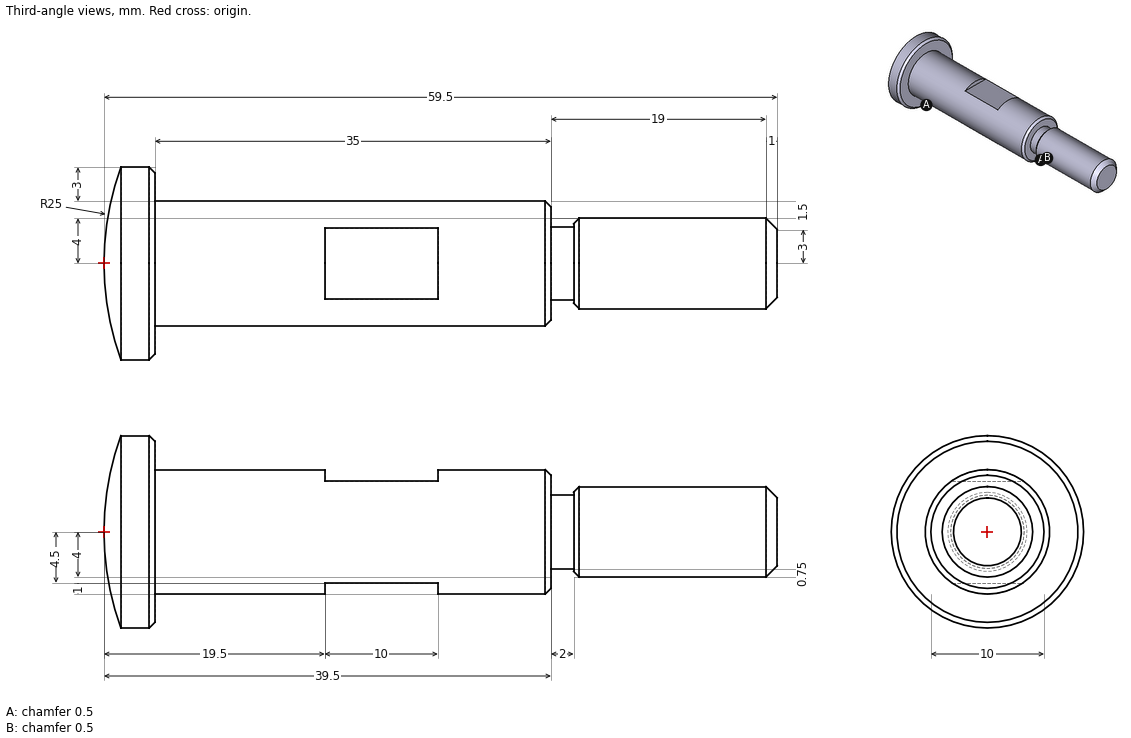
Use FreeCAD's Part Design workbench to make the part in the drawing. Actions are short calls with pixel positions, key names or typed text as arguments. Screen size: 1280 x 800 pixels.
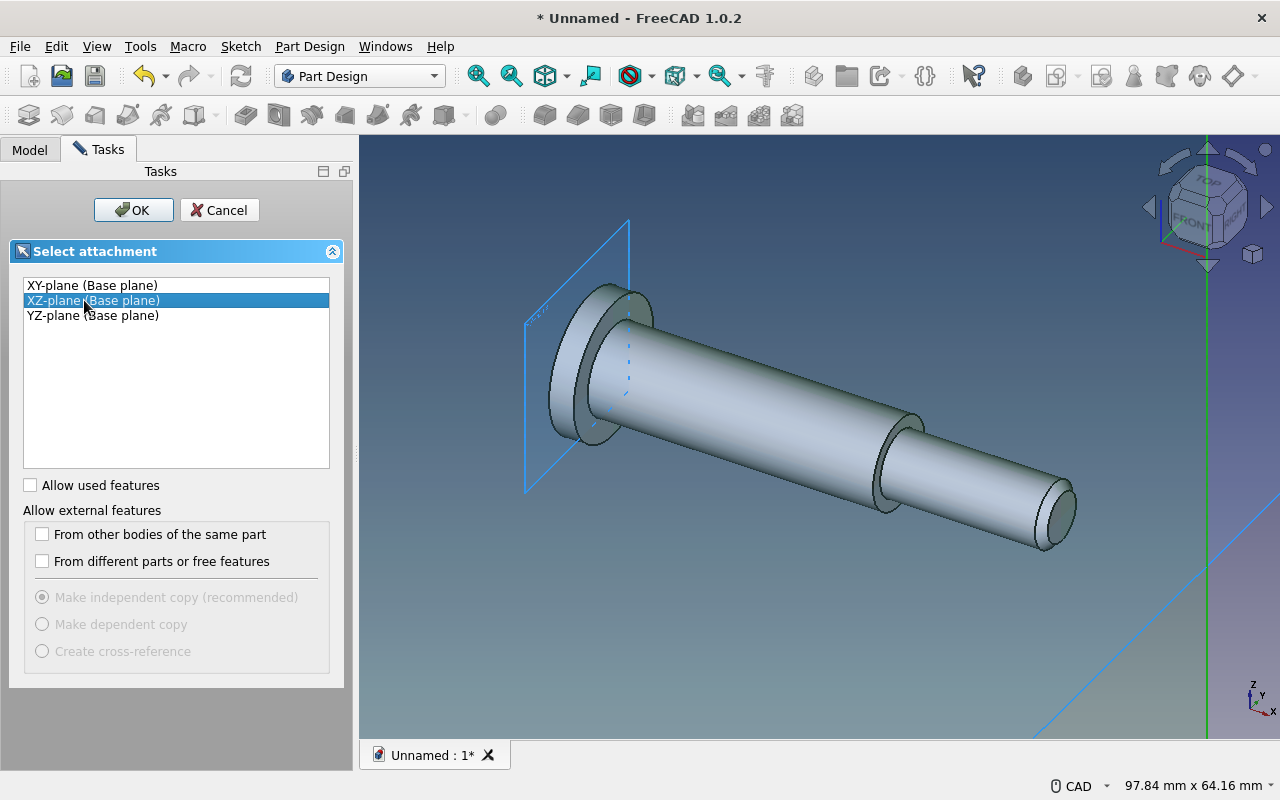
click(134, 210)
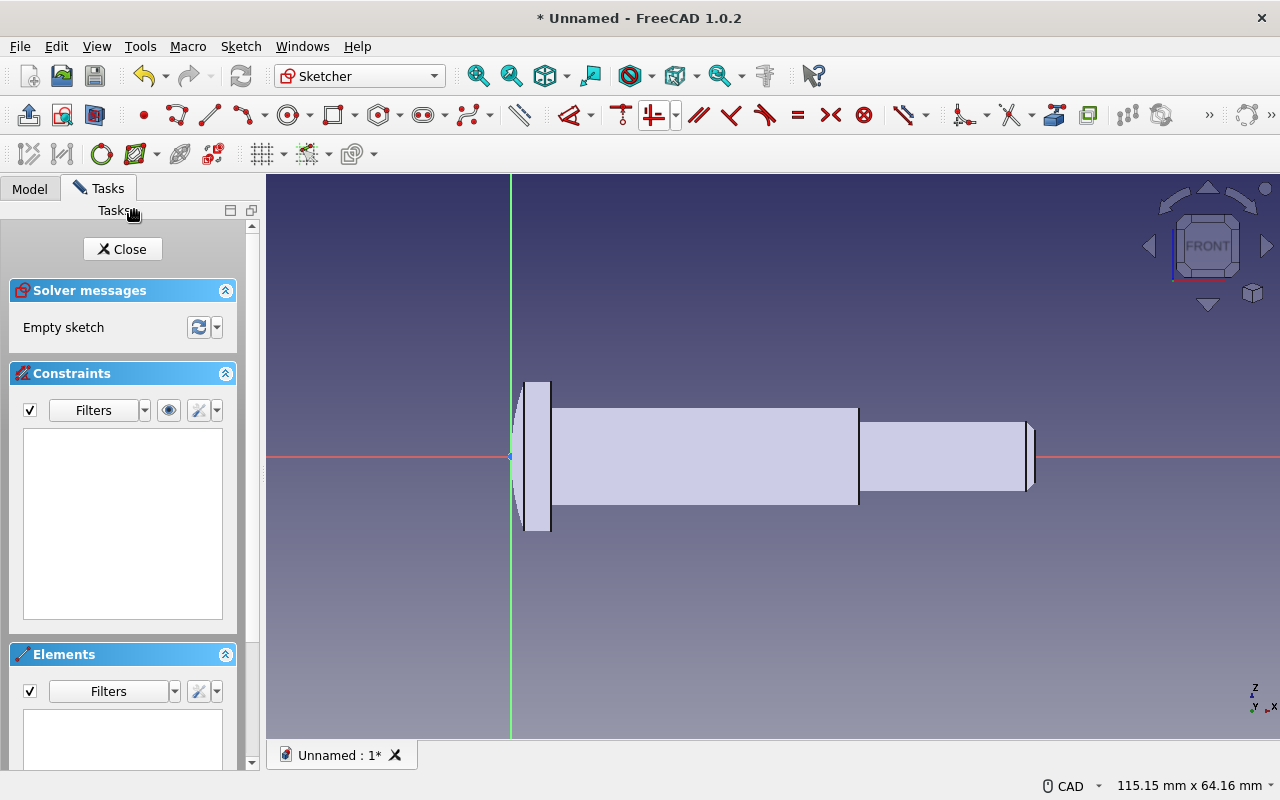
key(q)
key(s)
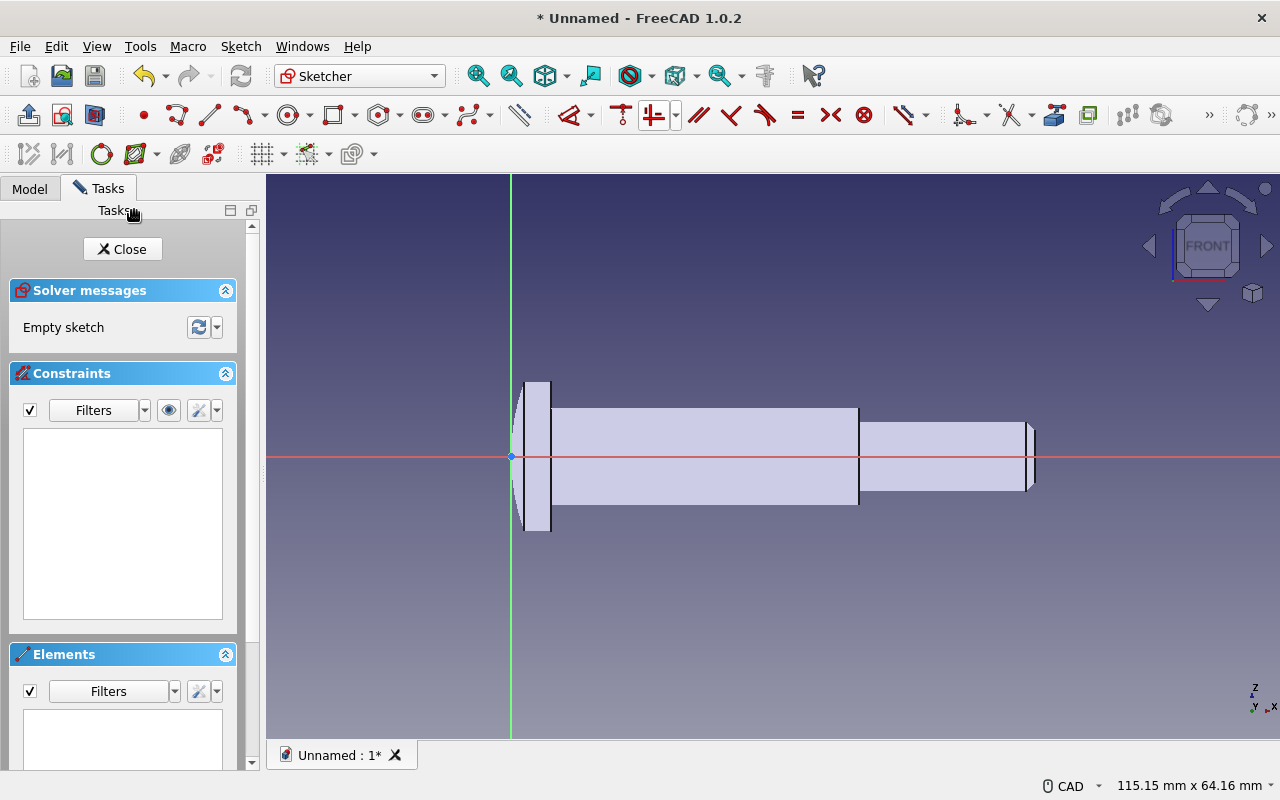
scroll(731, 509, up, 9)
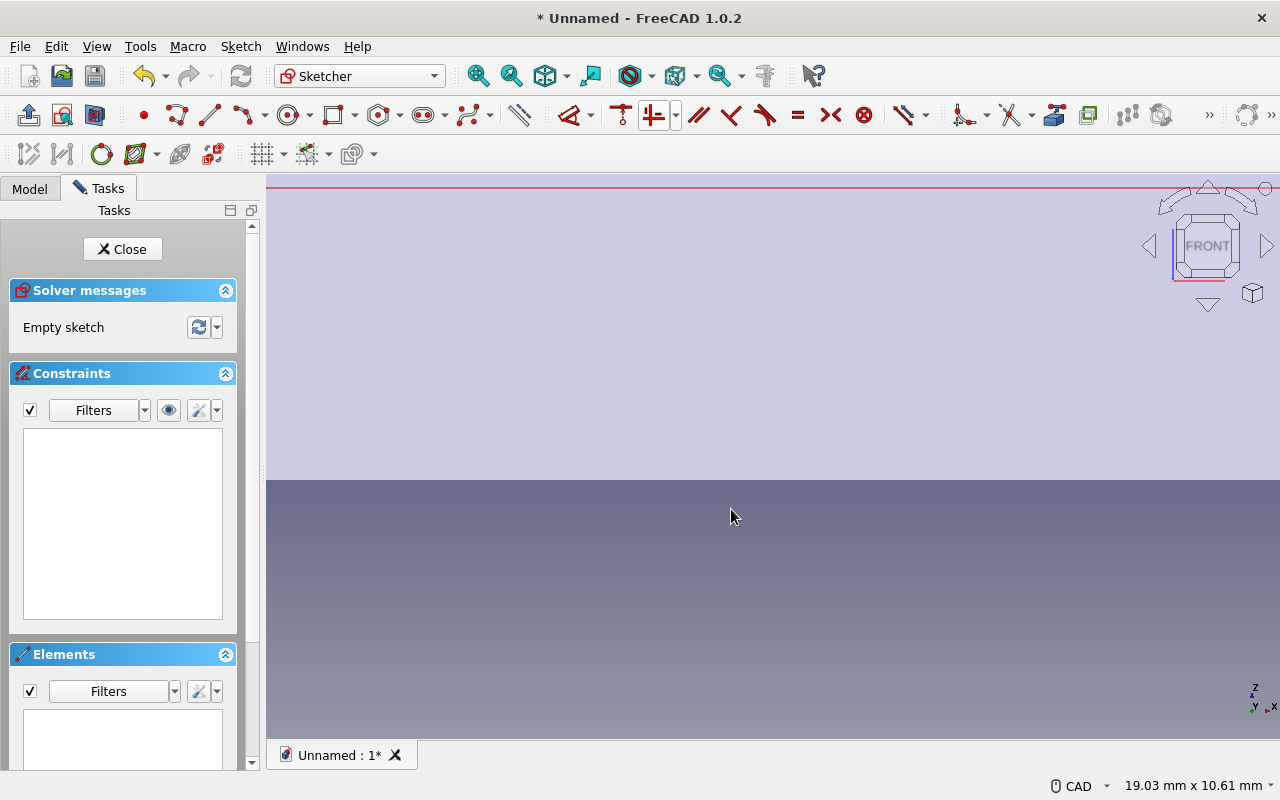
click(332, 116)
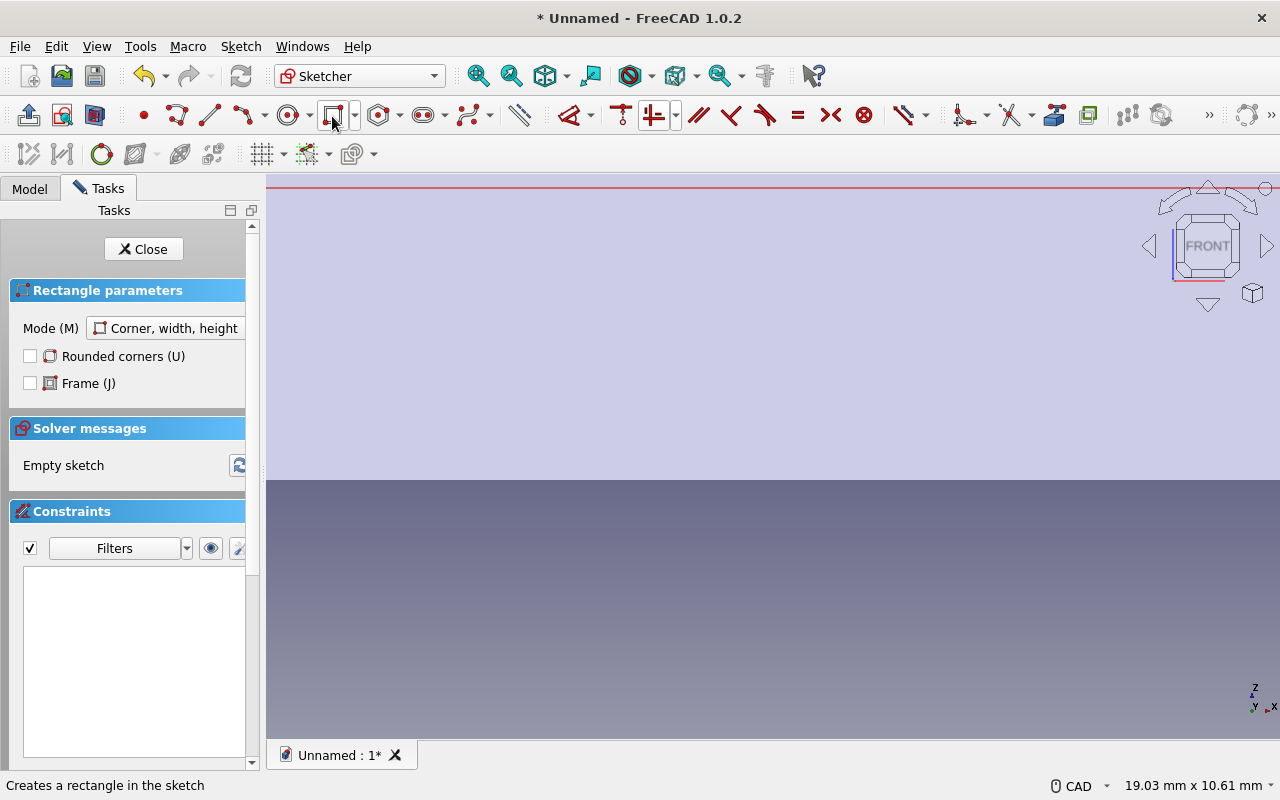
click(437, 428)
move(969, 481)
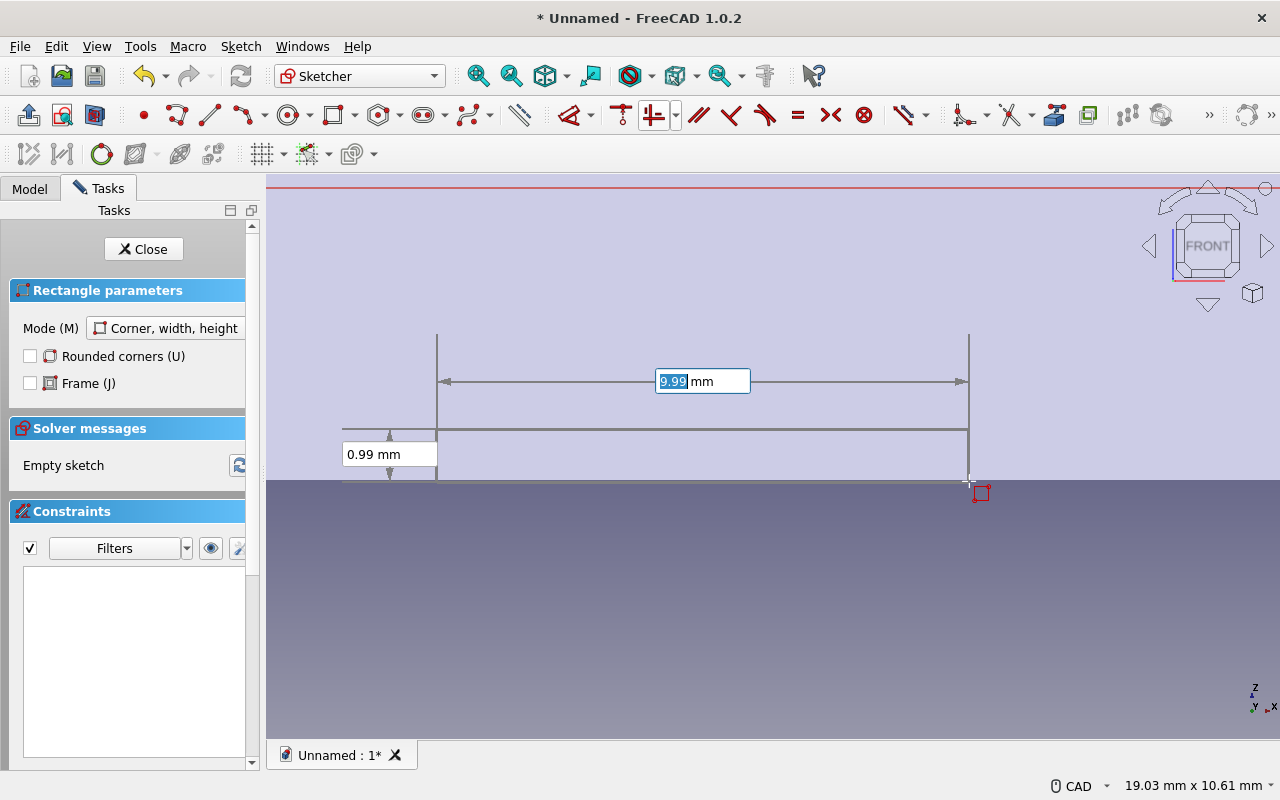
text(10)
key(Tab)
text(1)
key(Return)
key(Escape)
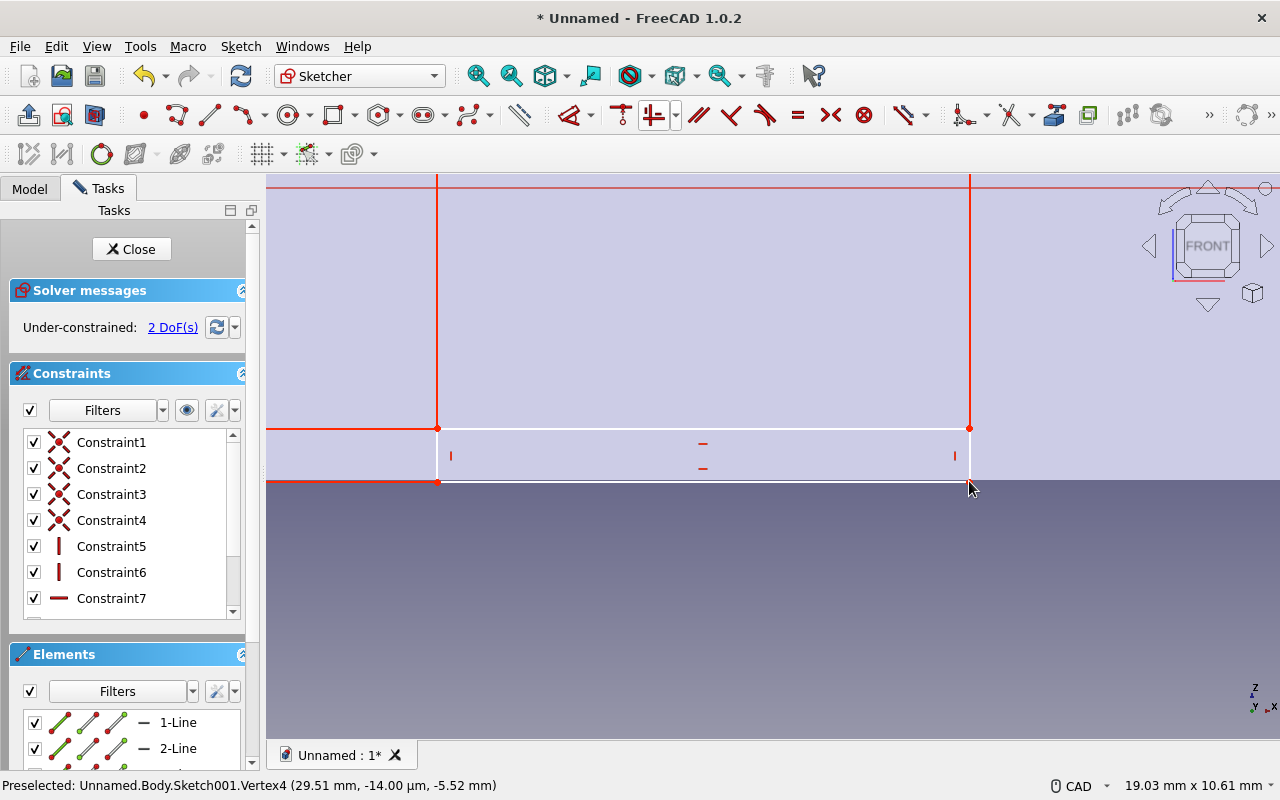
click(568, 116)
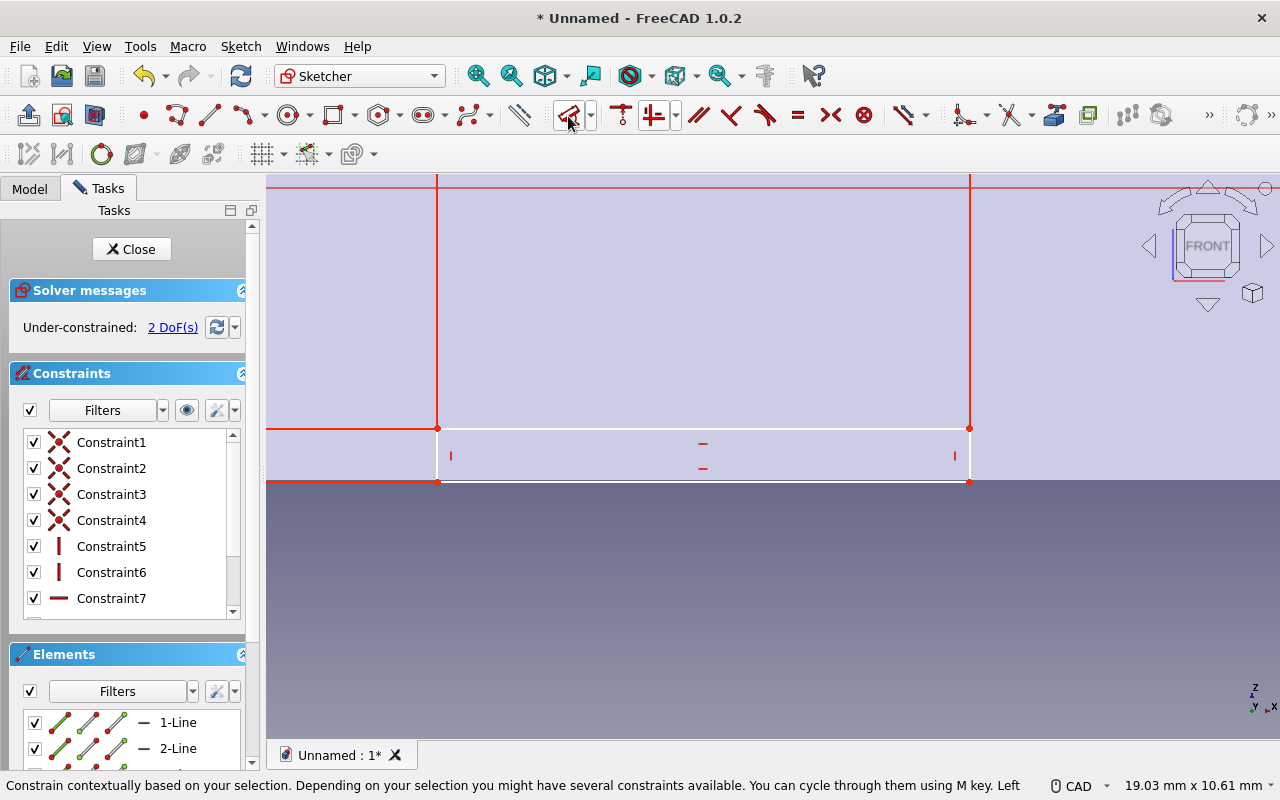
click(437, 429)
click(471, 315)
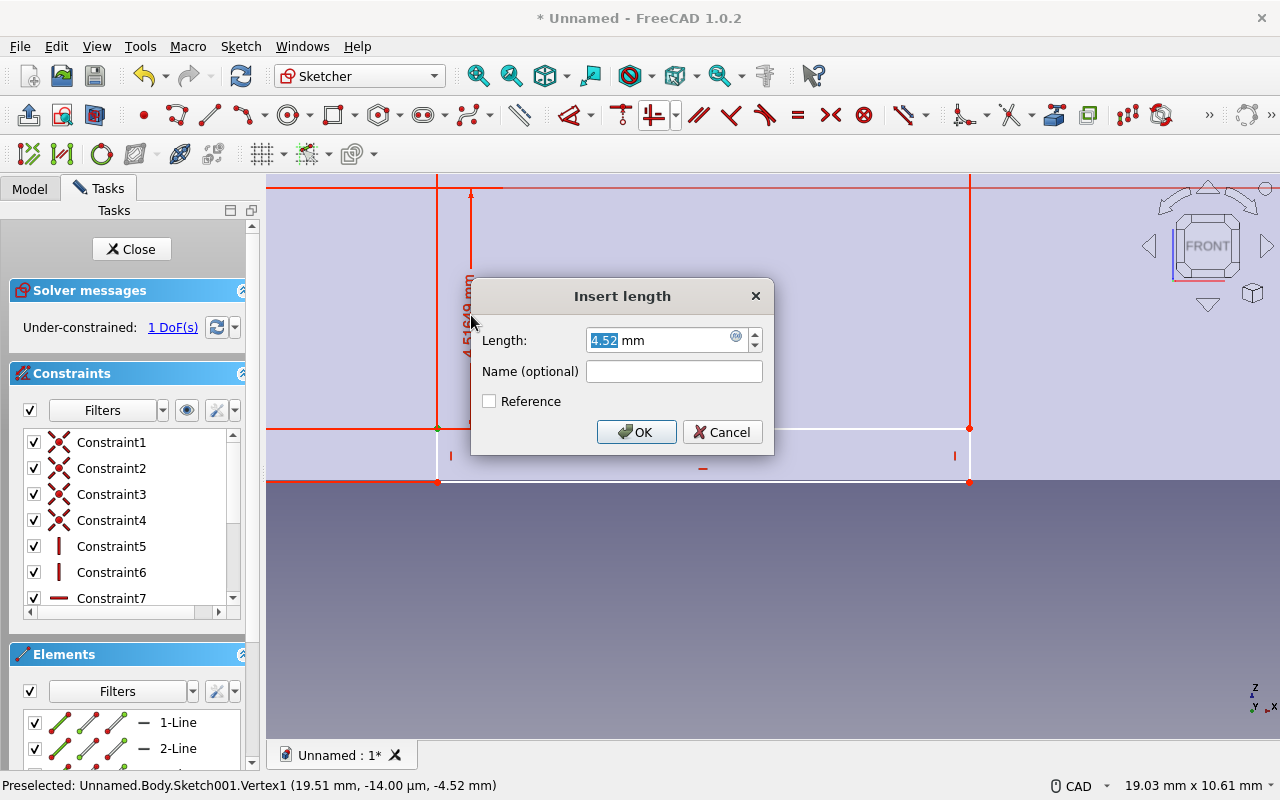
text(4.5)
key(Return)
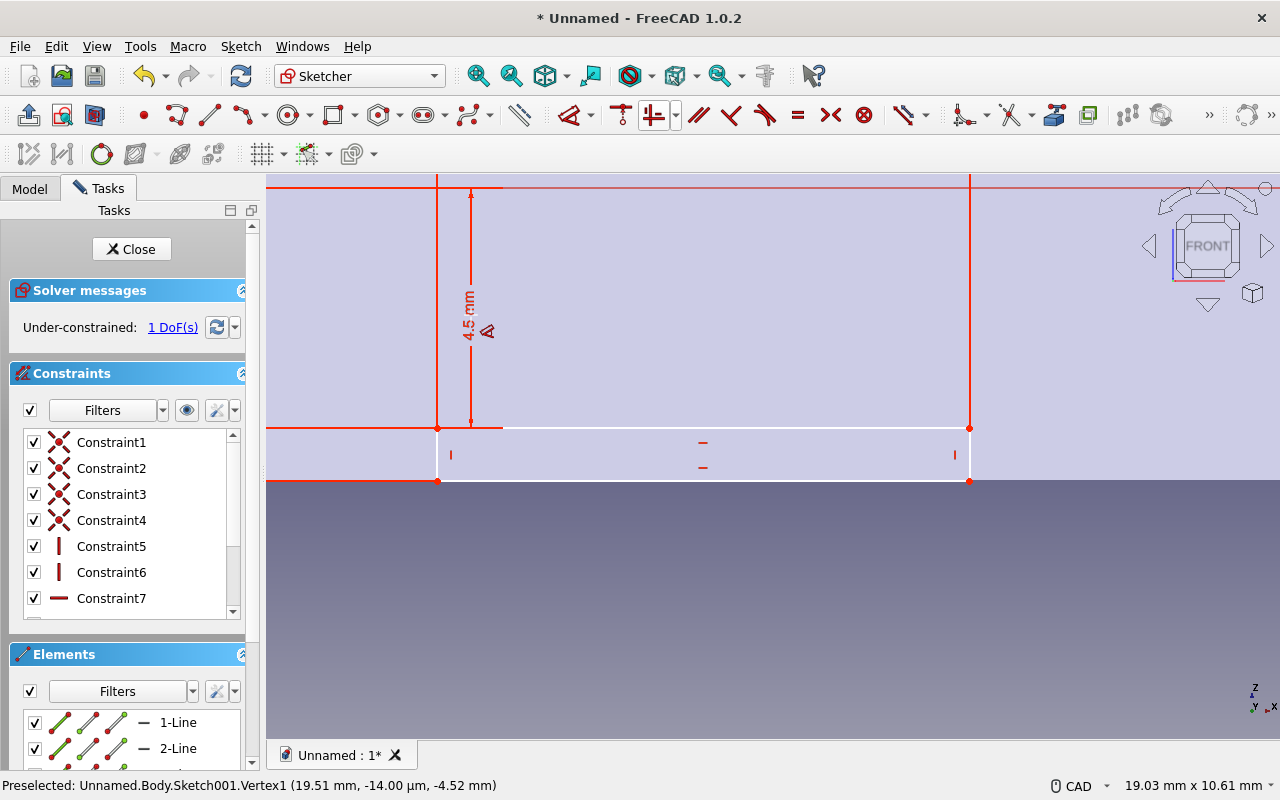
click(437, 428)
click(365, 462)